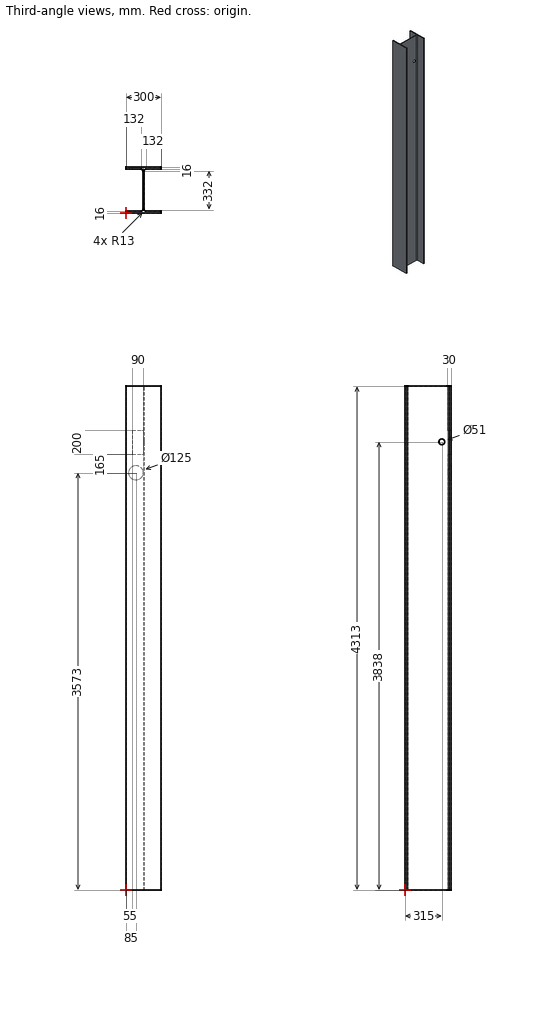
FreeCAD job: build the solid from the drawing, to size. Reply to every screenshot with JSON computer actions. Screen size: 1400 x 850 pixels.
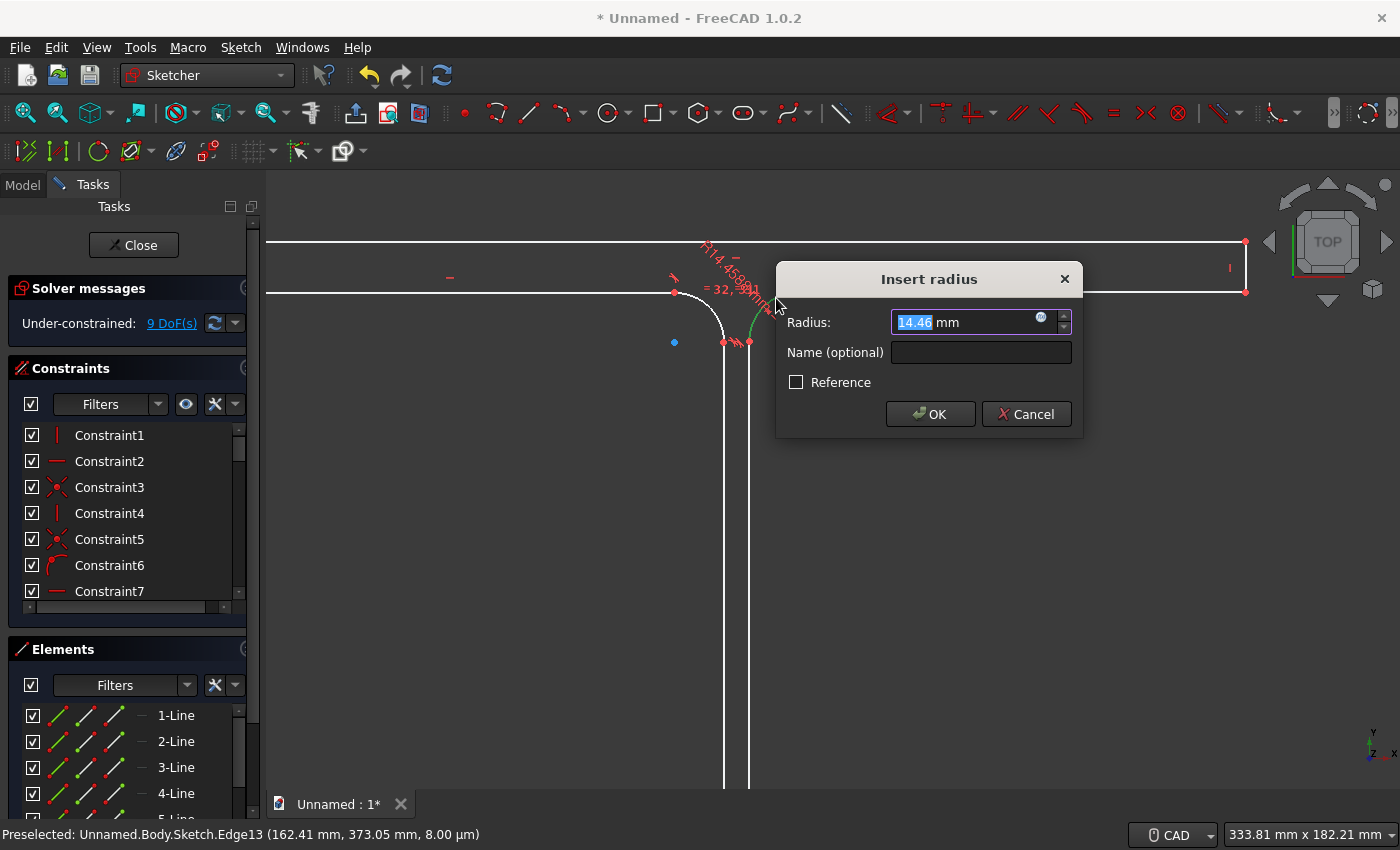
{"action": "type", "text": "13"}
{"action": "key", "text": "Return"}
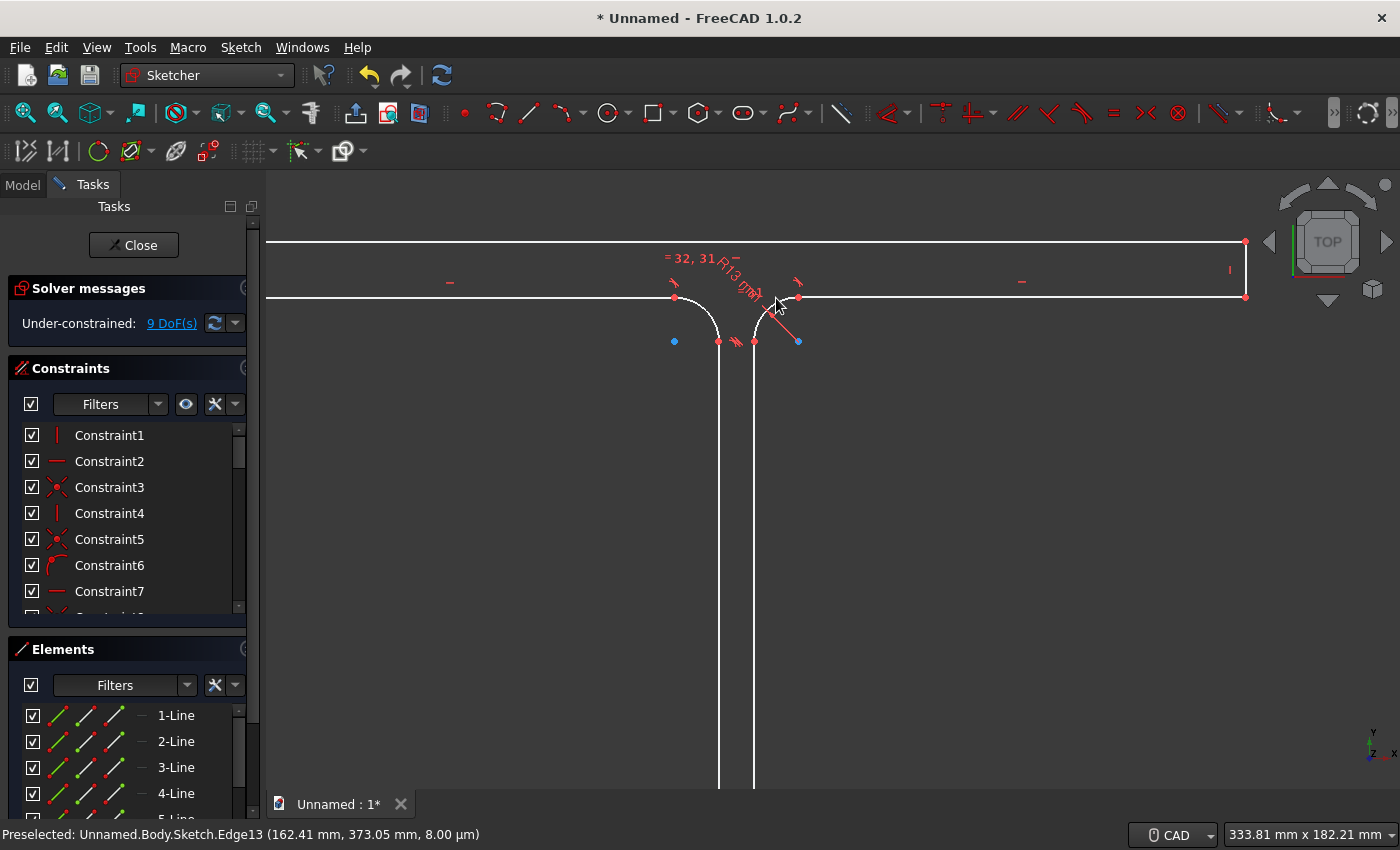
{"action": "scroll", "coordinate": [776, 298], "scroll_direction": "down", "scroll_amount": 6}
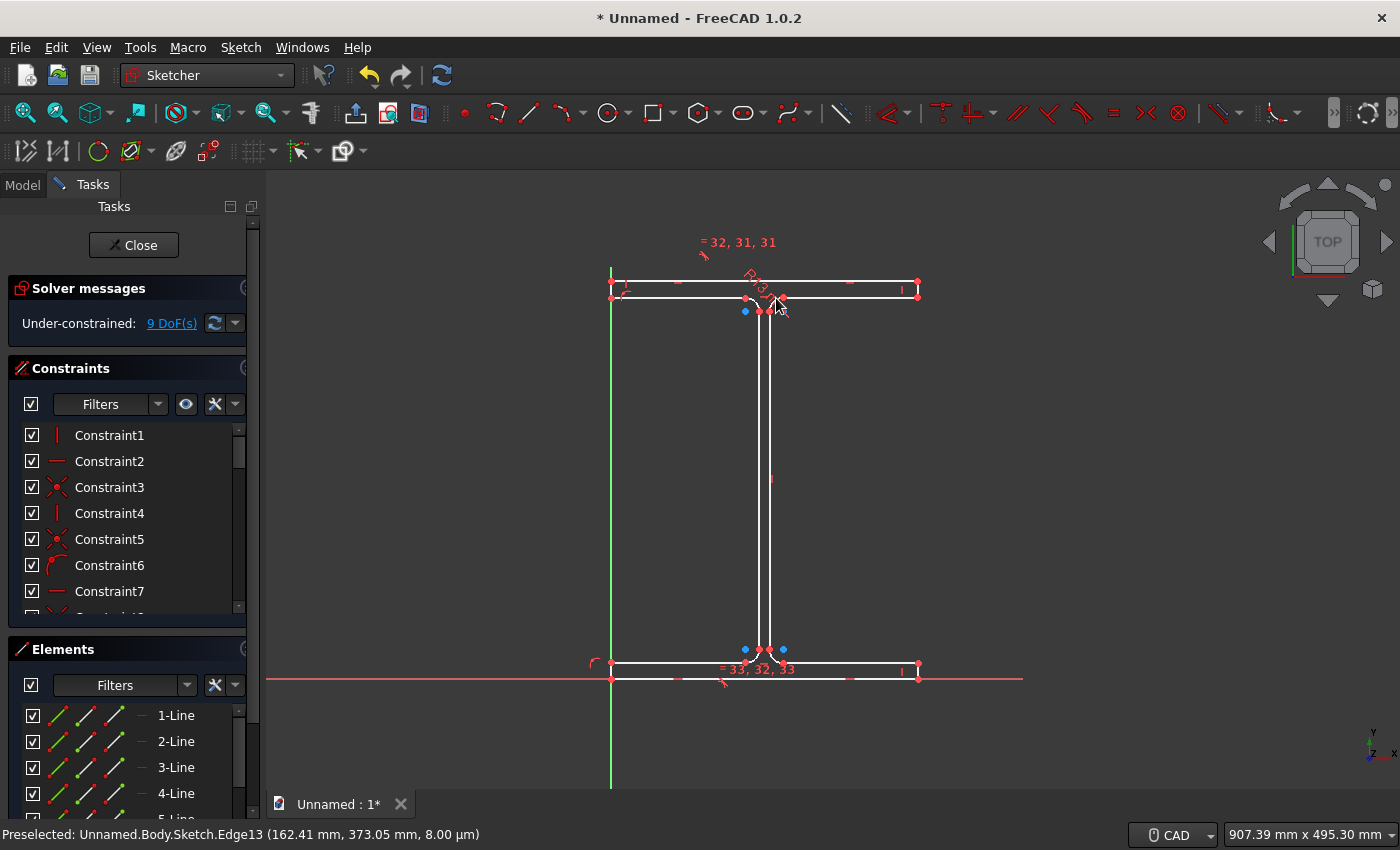
{"action": "scroll", "coordinate": [918, 293], "scroll_direction": "up", "scroll_amount": 6}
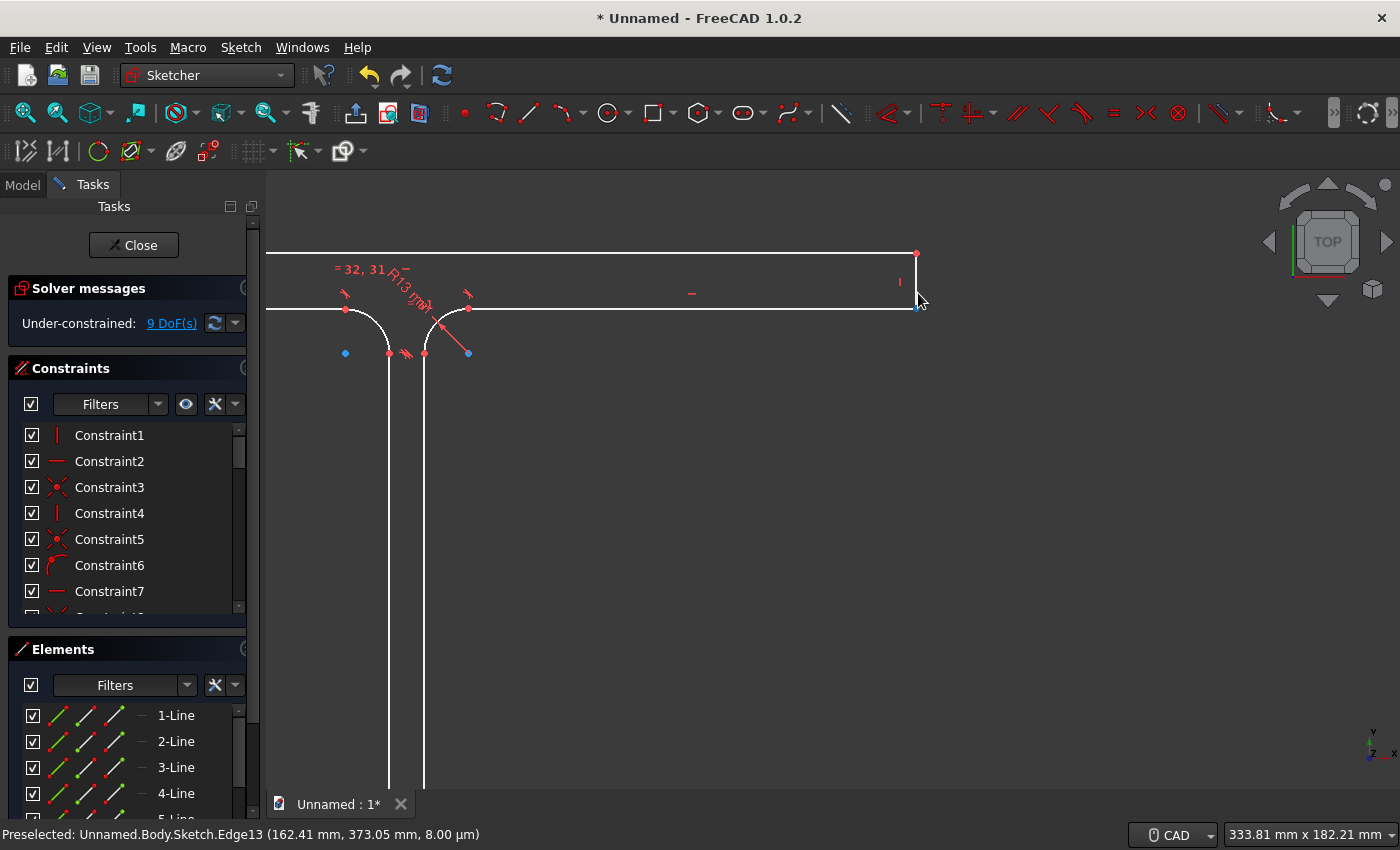
{"action": "left_click", "coordinate": [916, 292]}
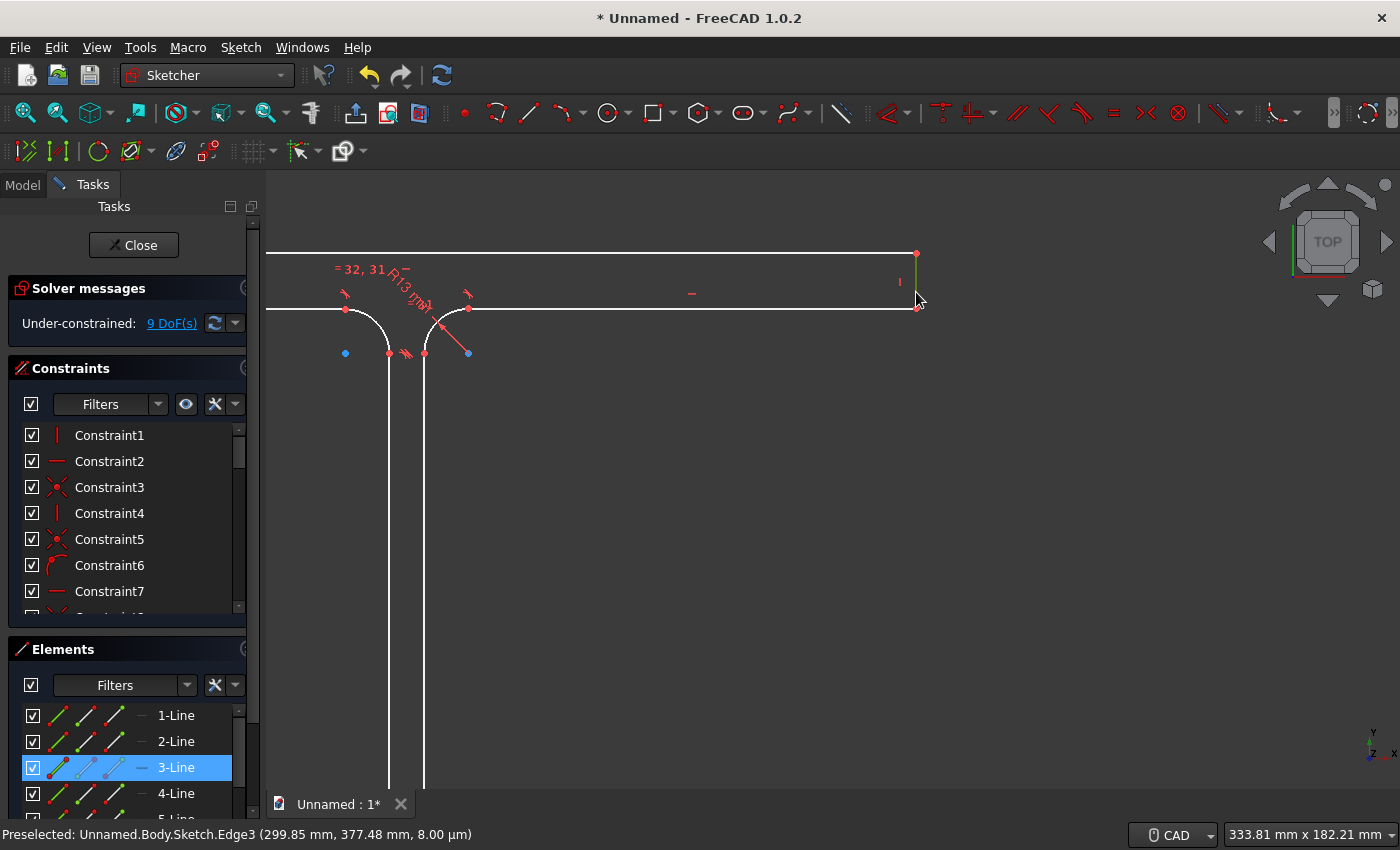
{"action": "key", "text": "i"}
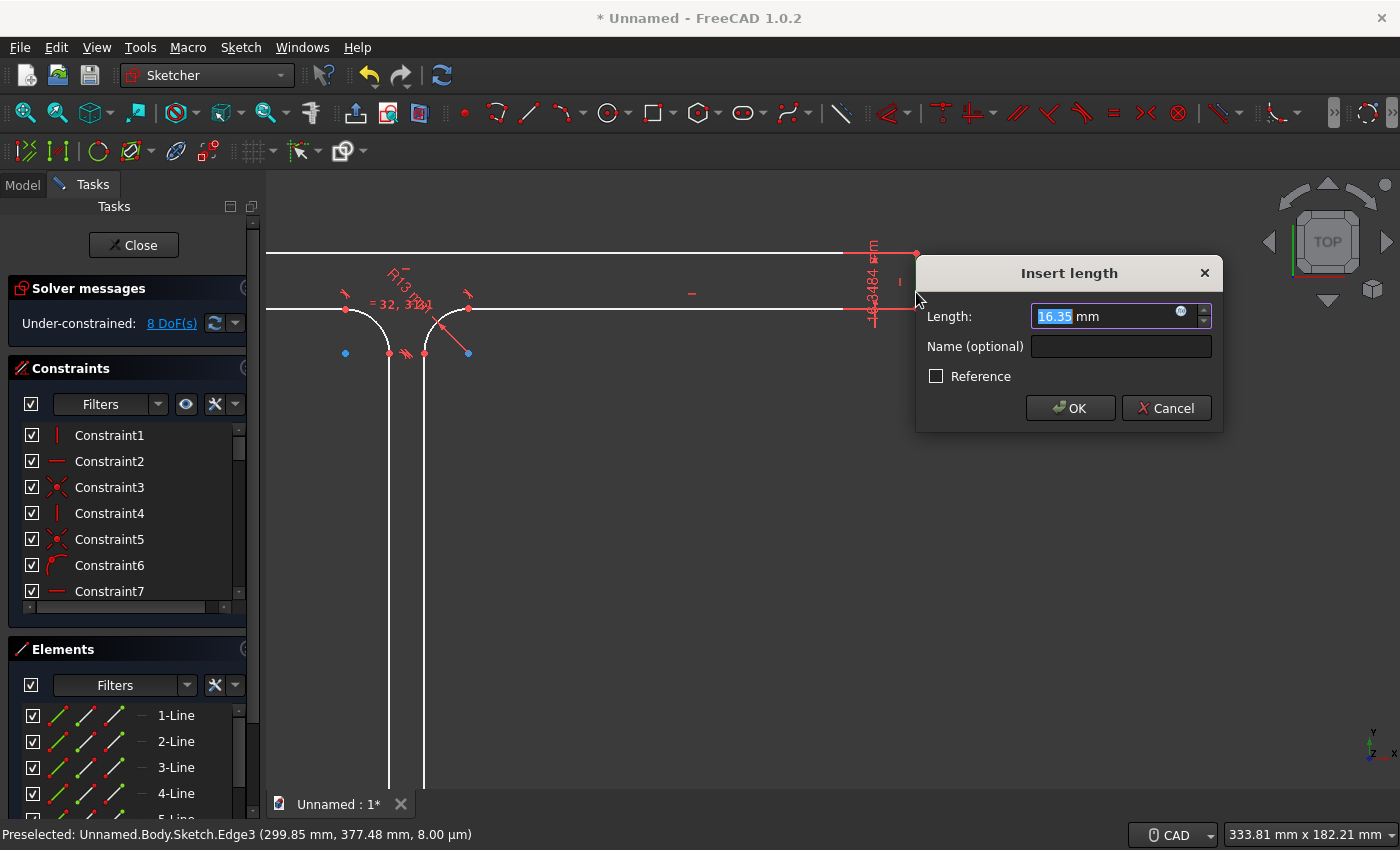
{"action": "type", "text": "16"}
{"action": "key", "text": "Return"}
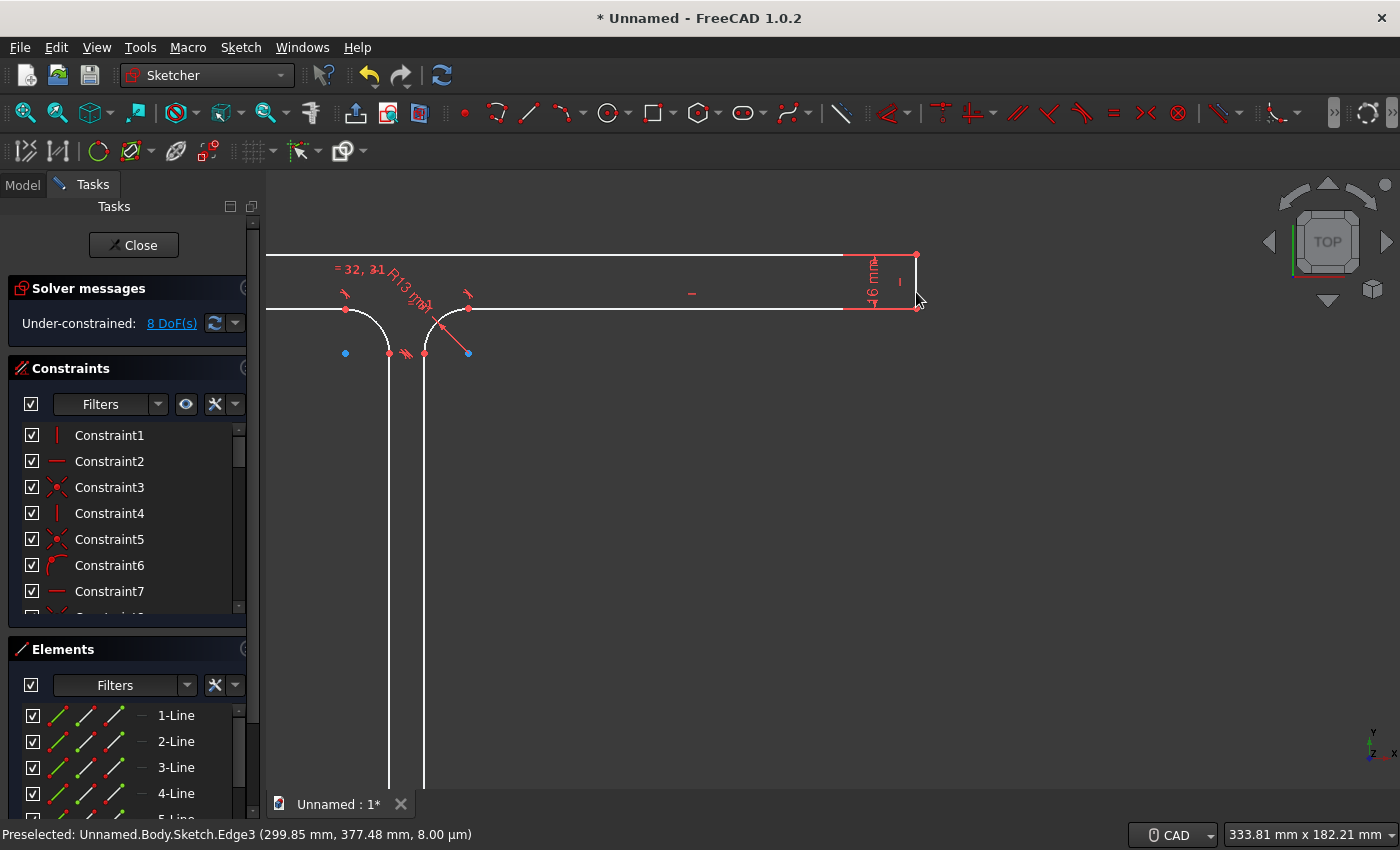
{"action": "scroll", "coordinate": [919, 293], "scroll_direction": "down", "scroll_amount": 6}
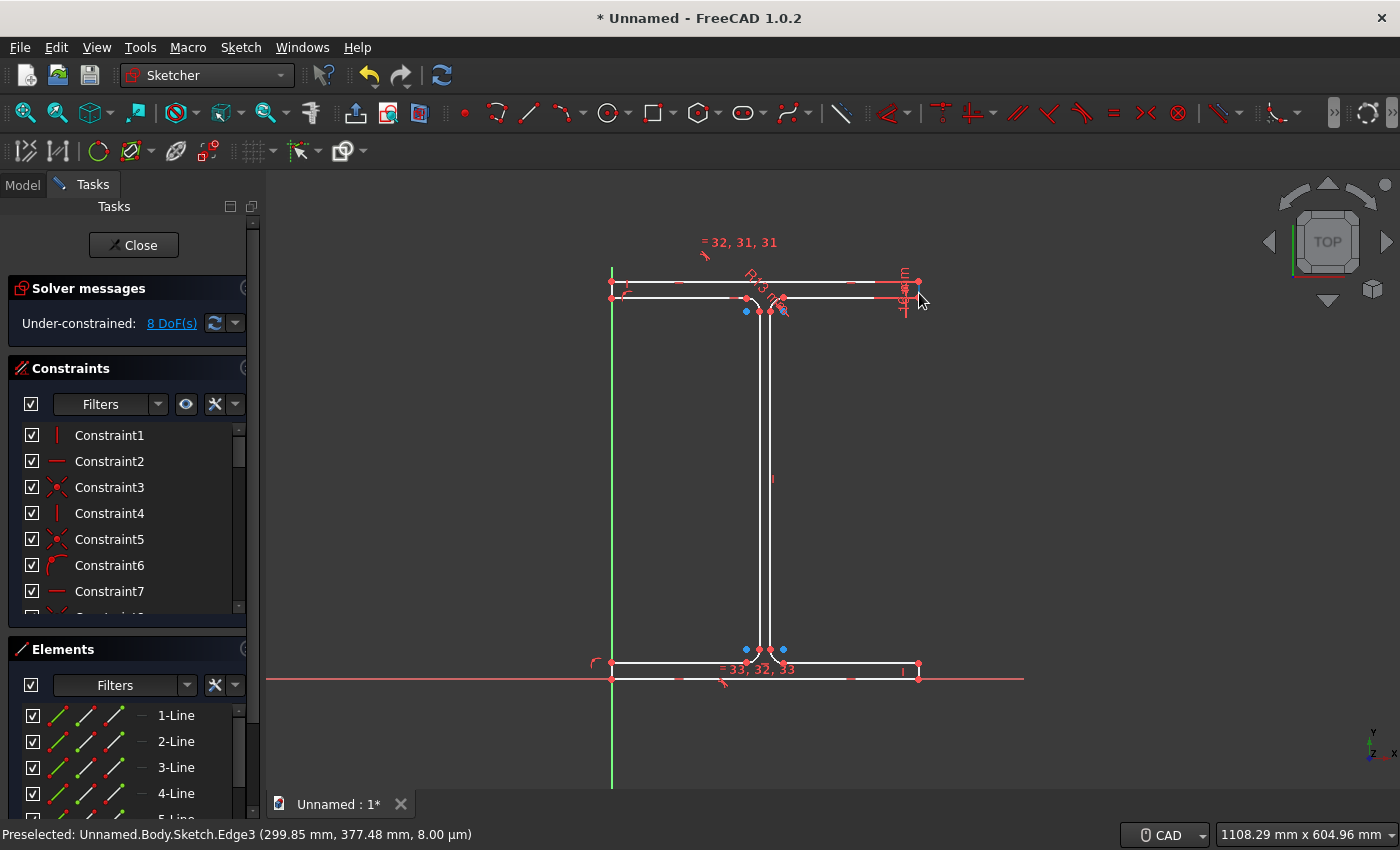
{"action": "scroll", "coordinate": [612, 287], "scroll_direction": "up", "scroll_amount": 6}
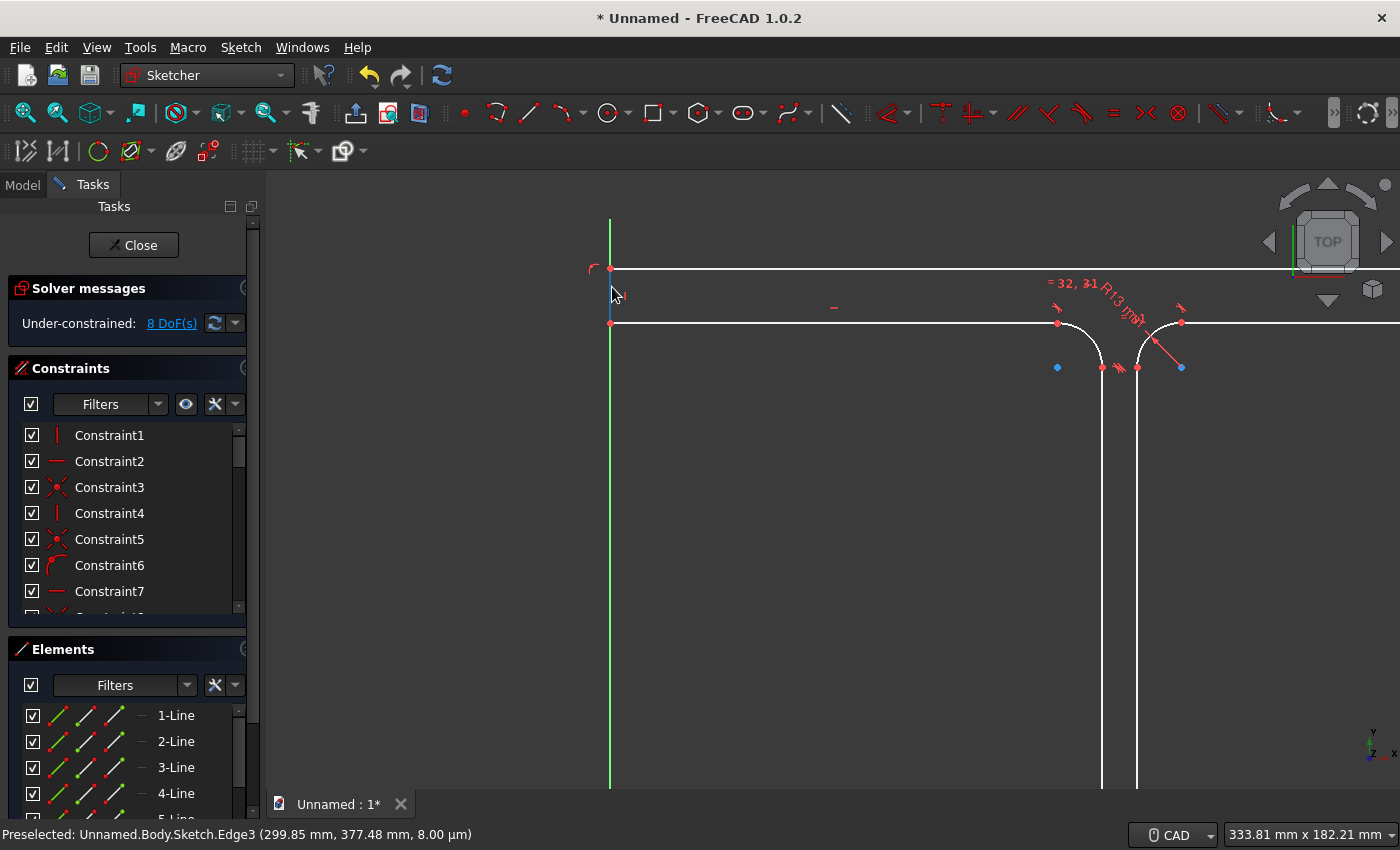
{"action": "left_click", "coordinate": [610, 285]}